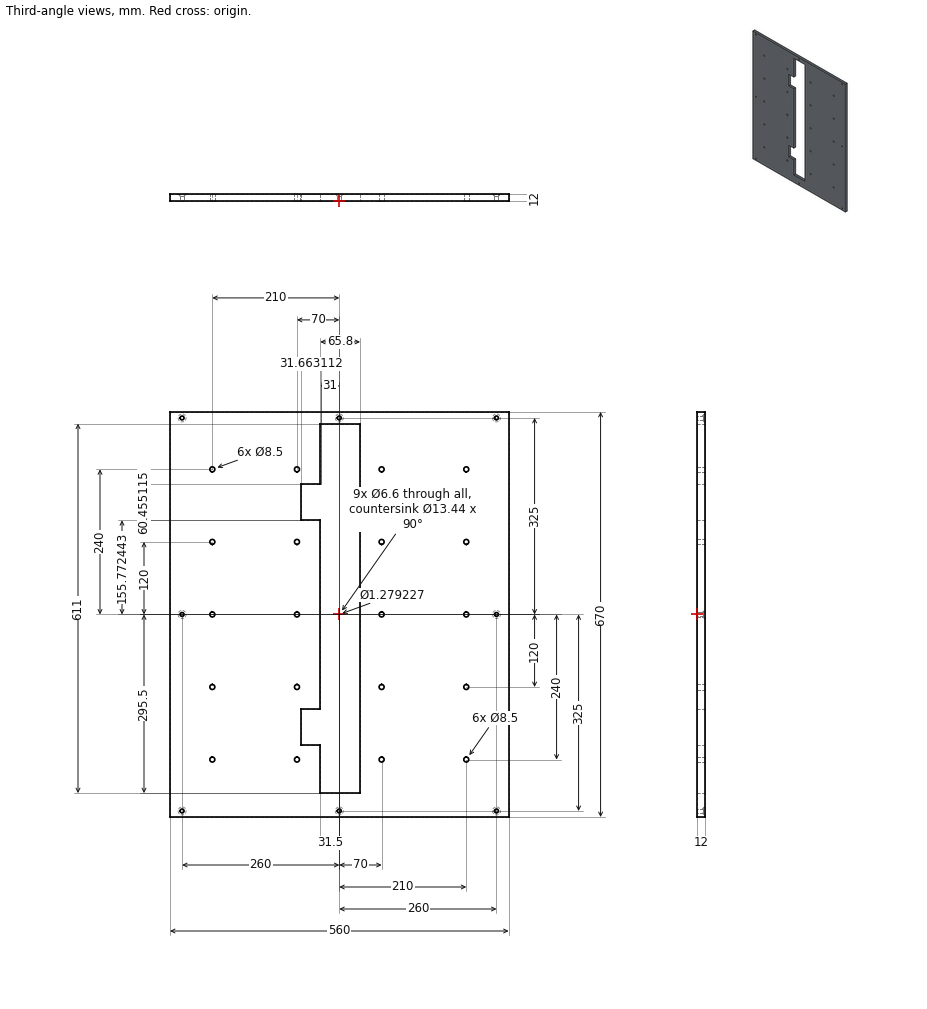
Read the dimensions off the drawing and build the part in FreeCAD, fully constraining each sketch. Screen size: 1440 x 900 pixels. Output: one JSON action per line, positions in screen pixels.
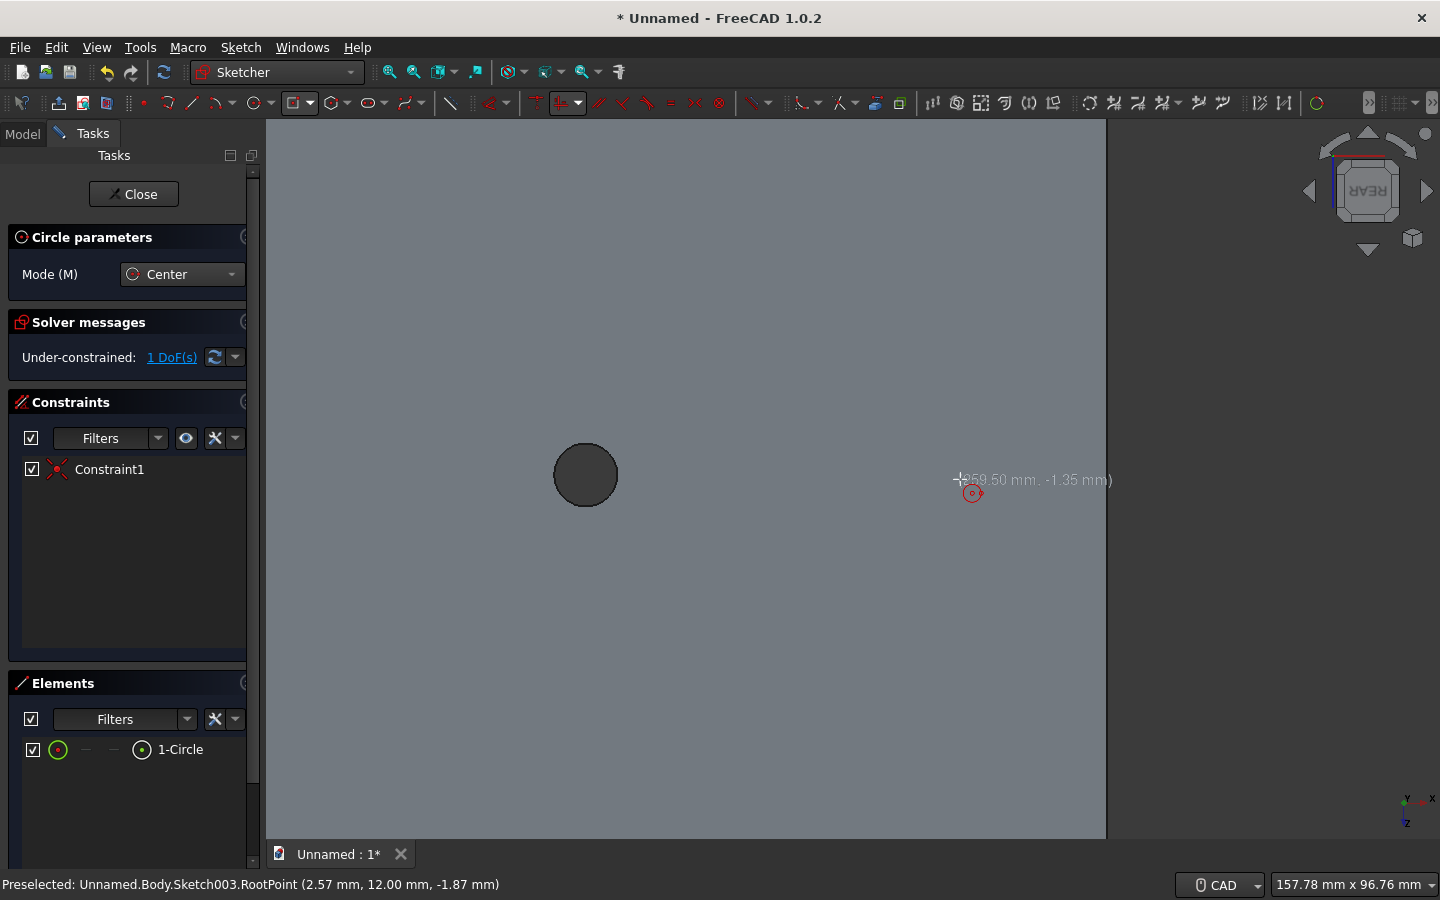
{"action": "scroll", "coordinate": [960, 479], "scroll_direction": "down", "scroll_amount": 12}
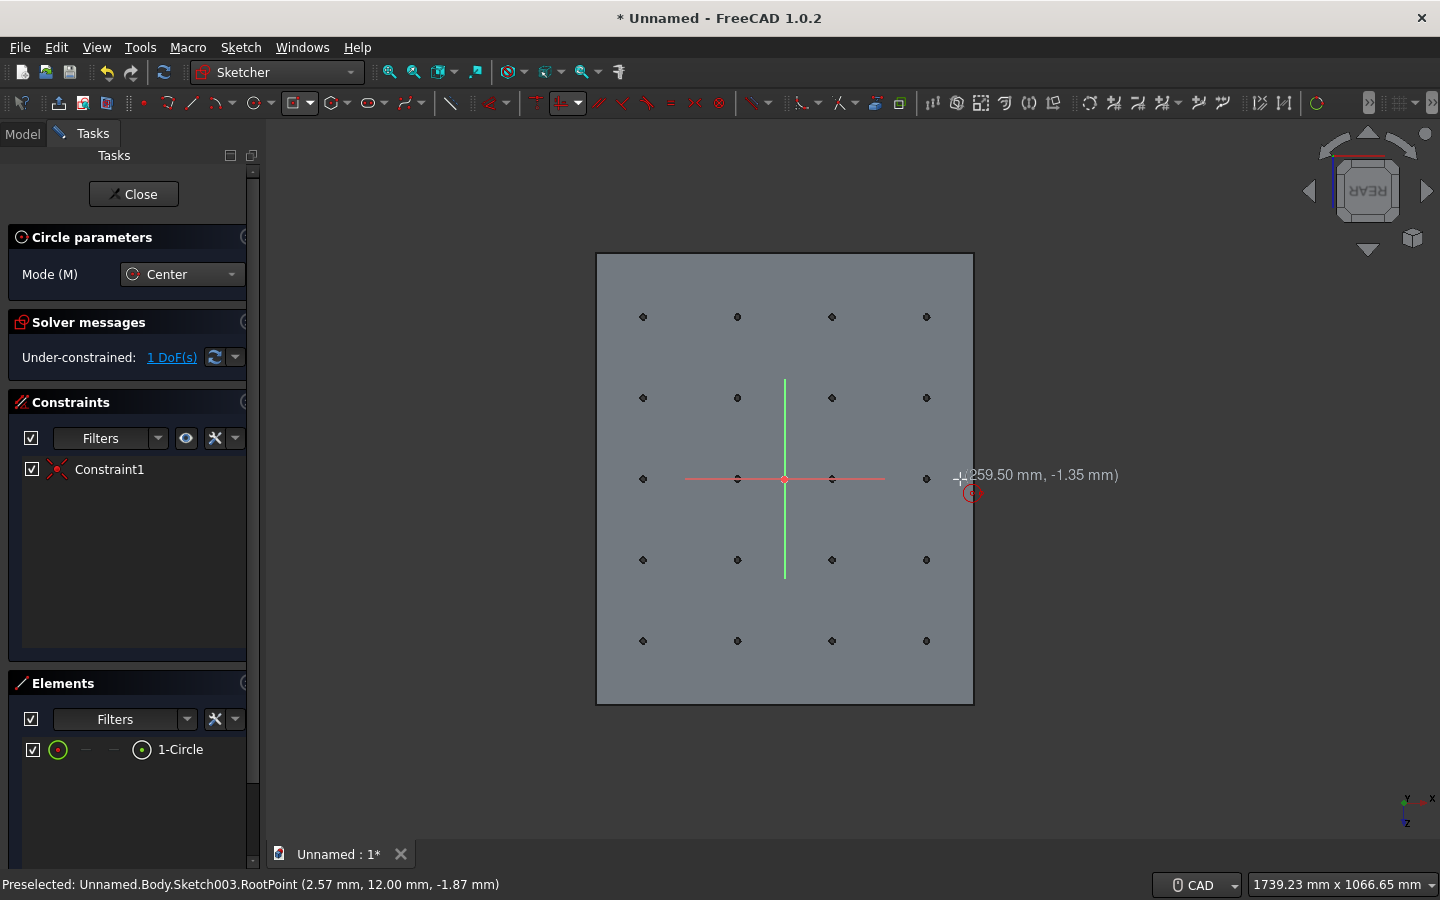
{"action": "left_click", "coordinate": [960, 479]}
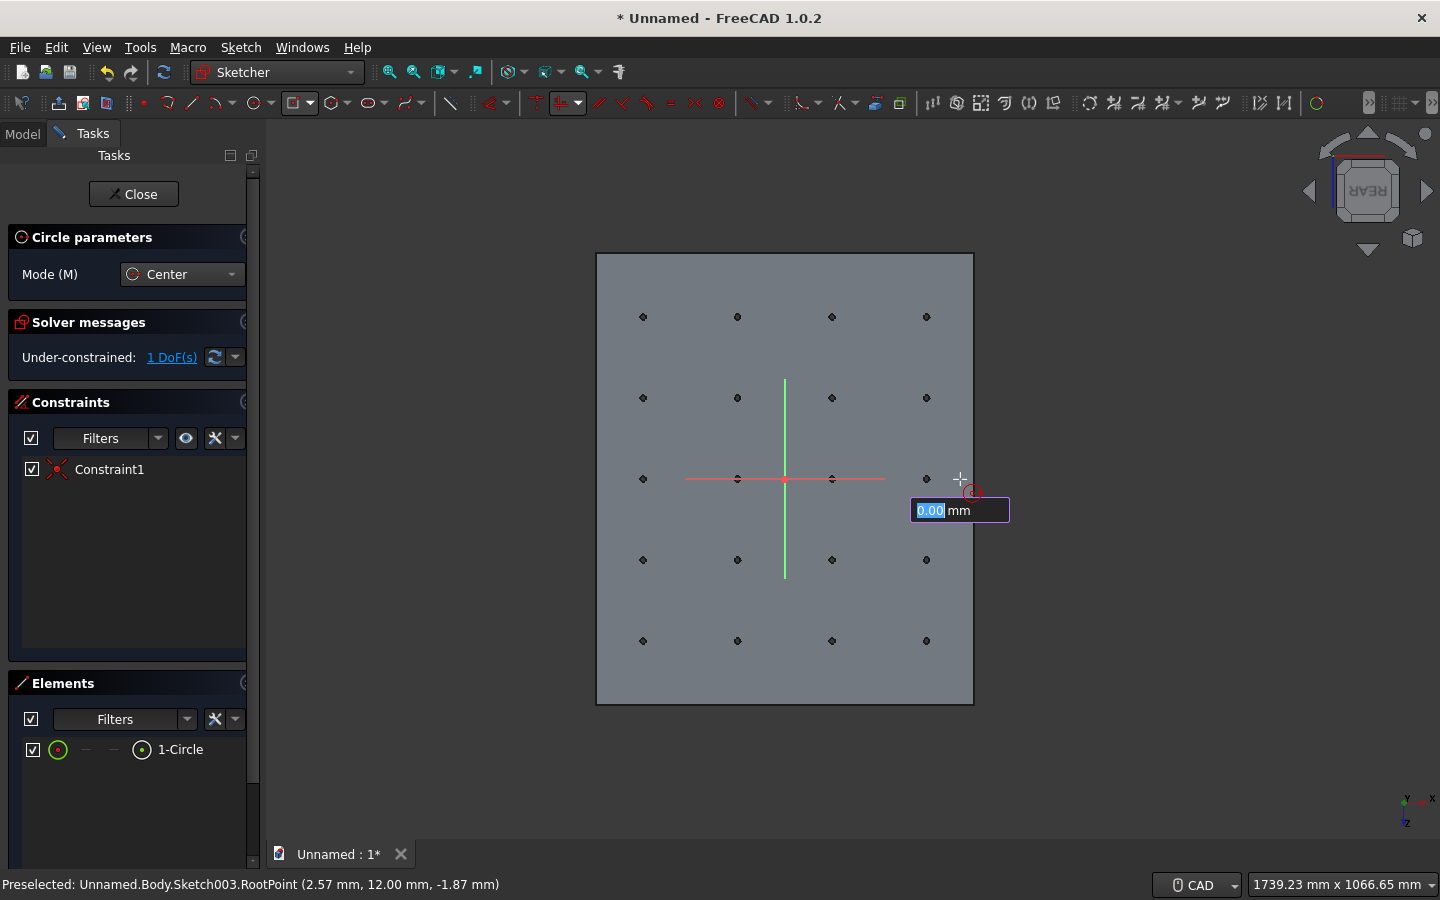
{"action": "scroll", "coordinate": [961, 477], "scroll_direction": "up", "scroll_amount": 11}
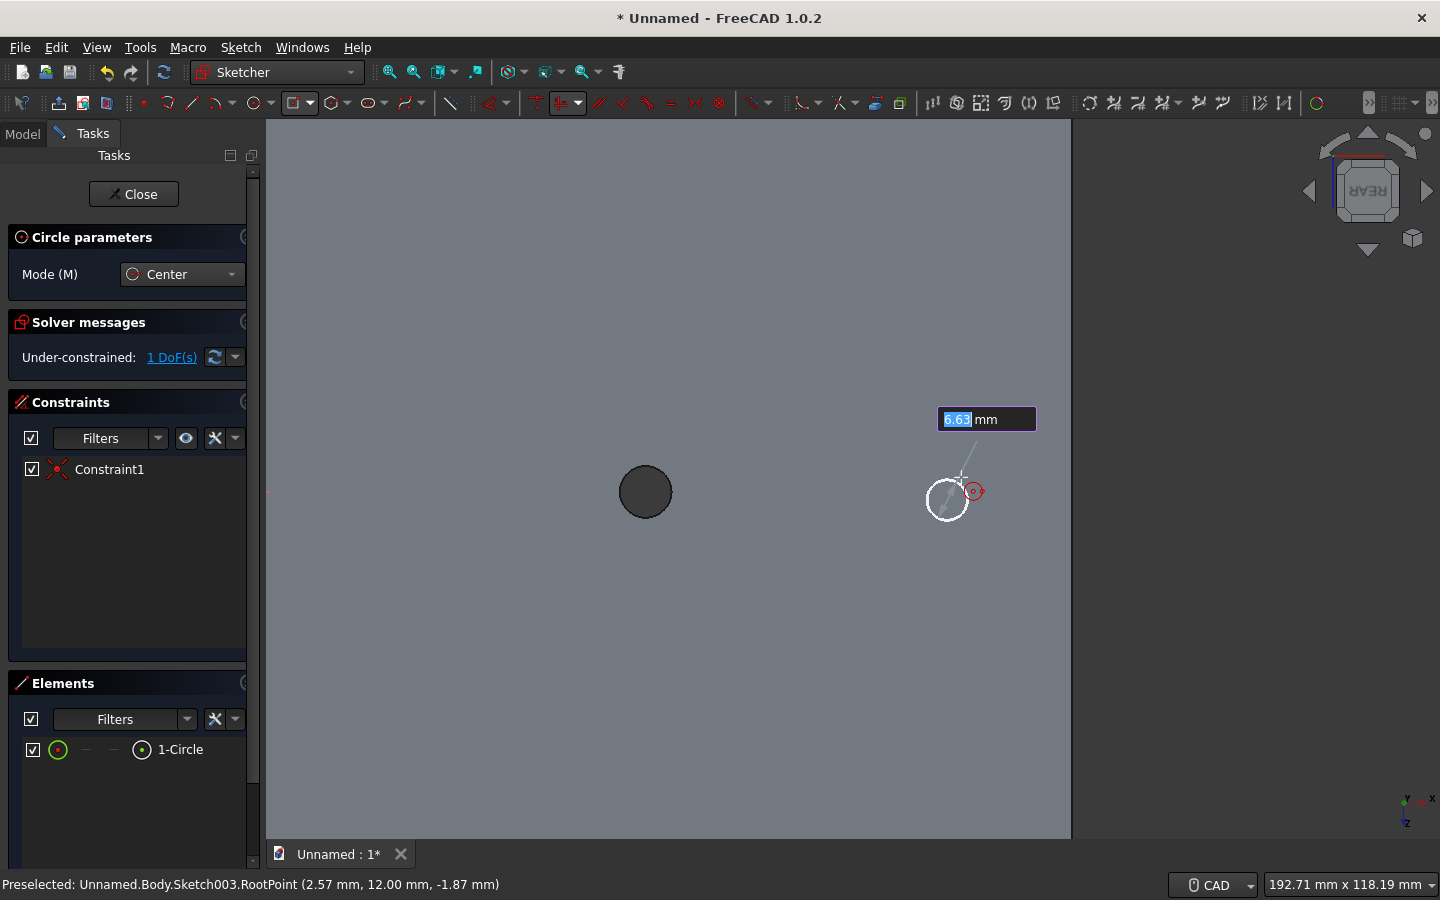
{"action": "left_click", "coordinate": [957, 473]}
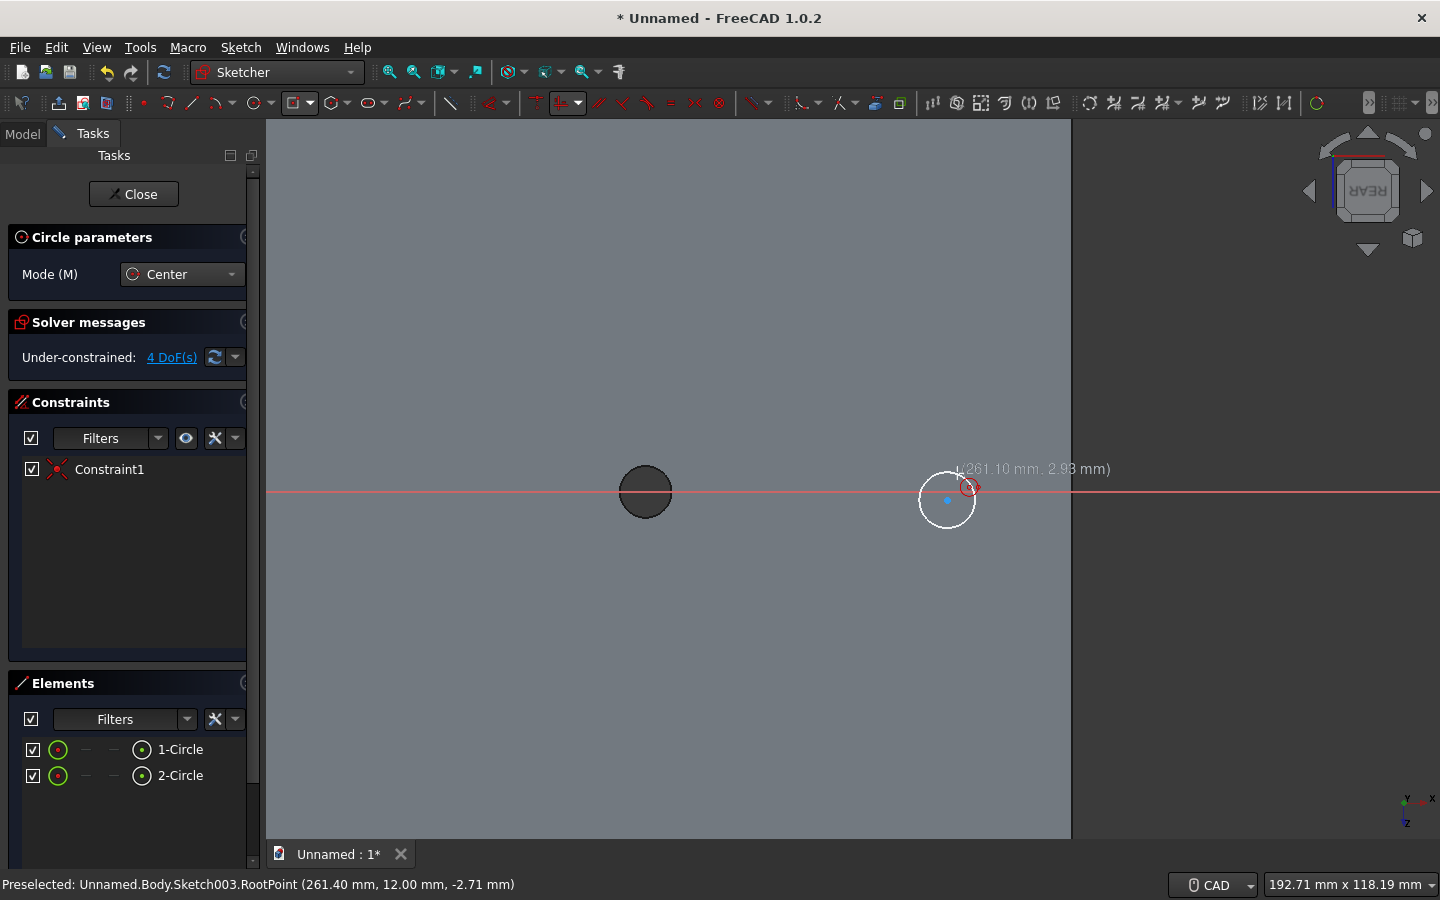
{"action": "scroll", "coordinate": [961, 477], "scroll_direction": "down", "scroll_amount": 11}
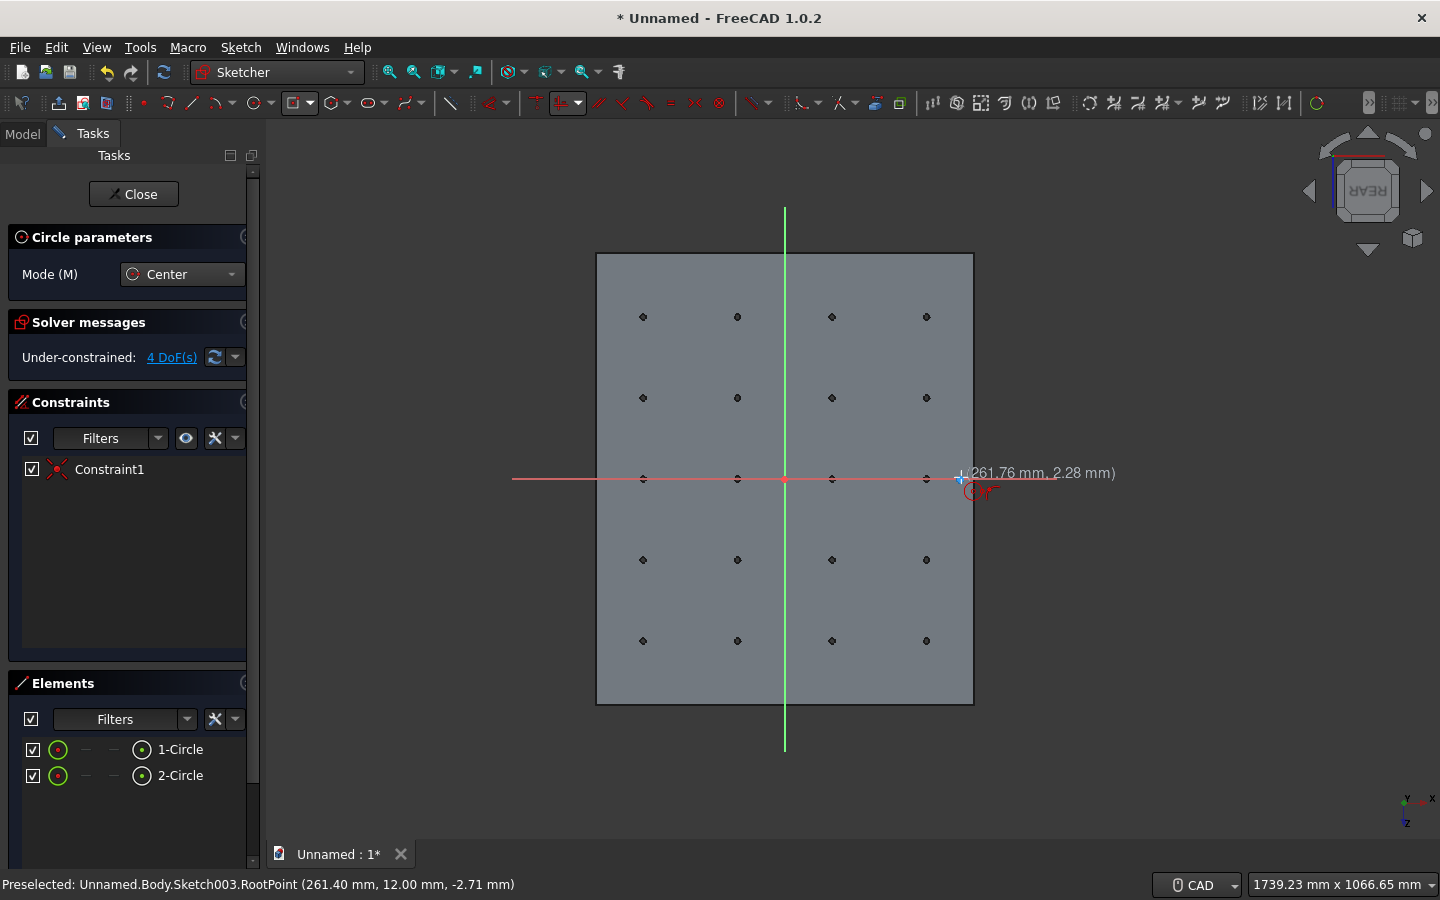
{"action": "scroll", "coordinate": [785, 260], "scroll_direction": "up", "scroll_amount": 12}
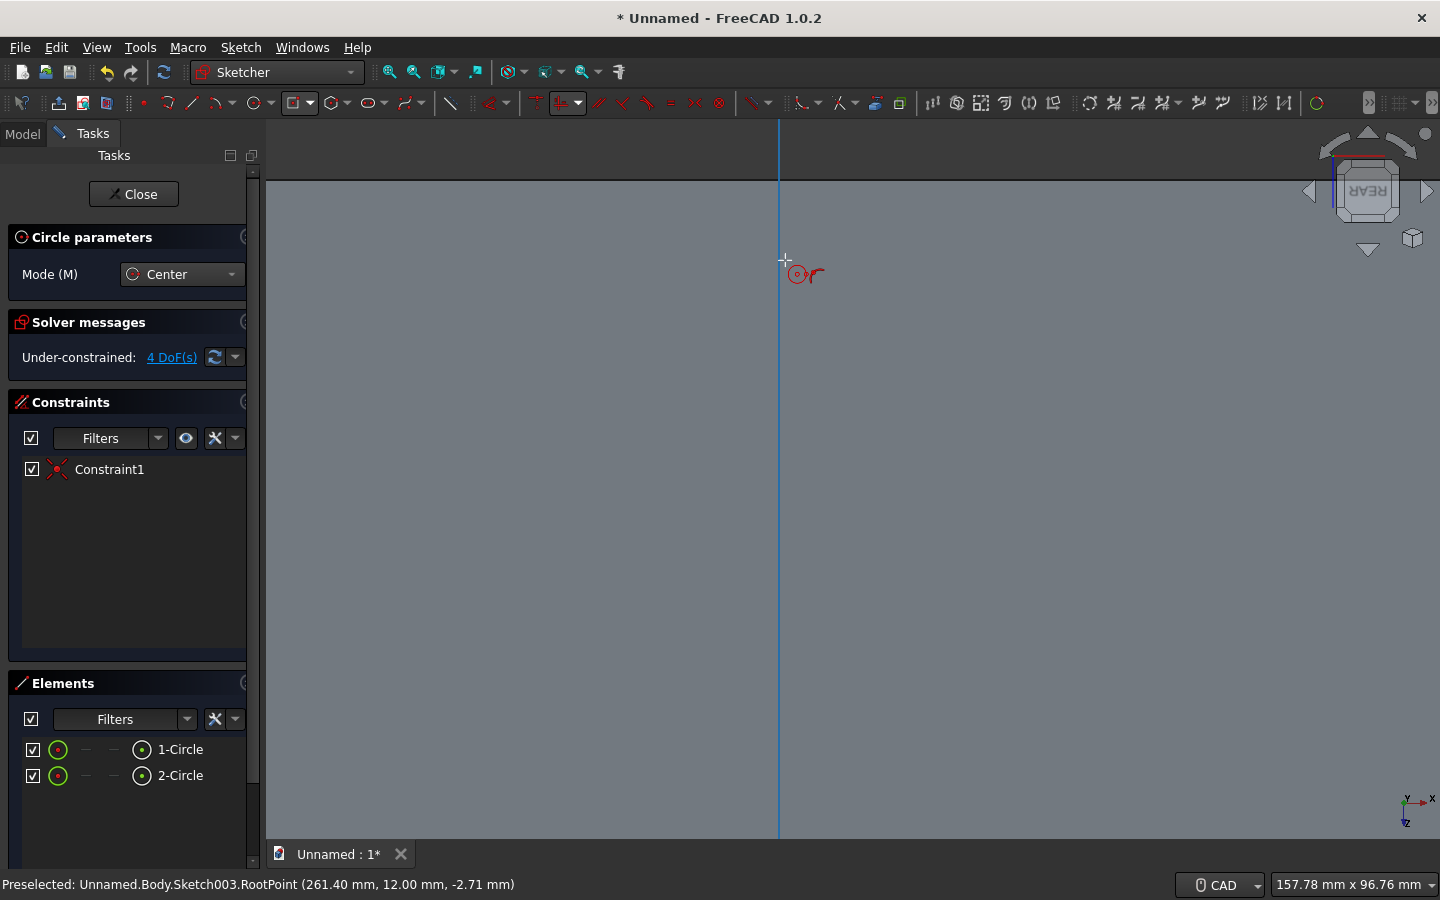
{"action": "scroll", "coordinate": [785, 260], "scroll_direction": "down", "scroll_amount": 12}